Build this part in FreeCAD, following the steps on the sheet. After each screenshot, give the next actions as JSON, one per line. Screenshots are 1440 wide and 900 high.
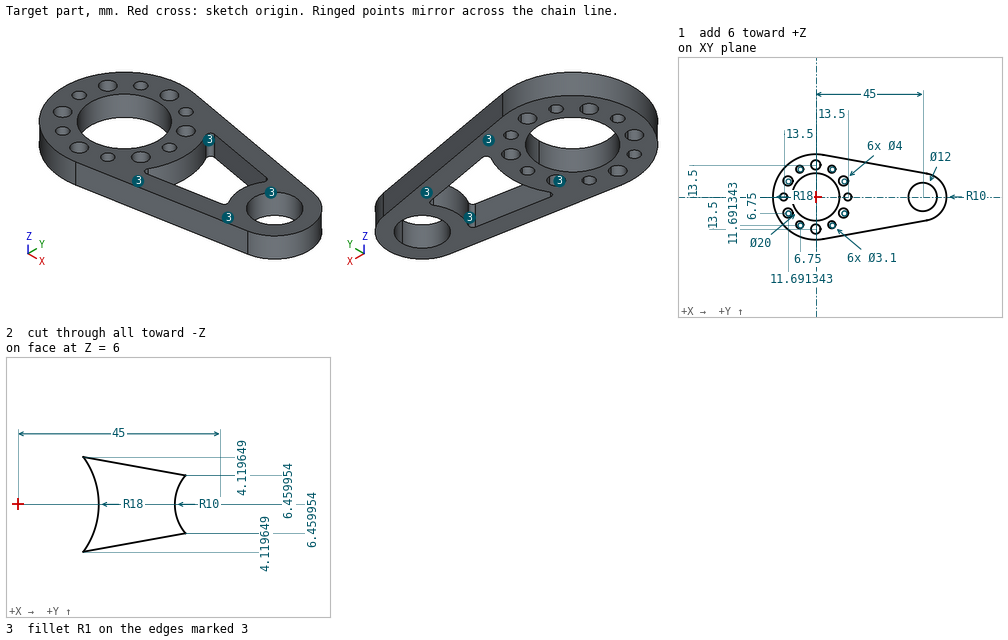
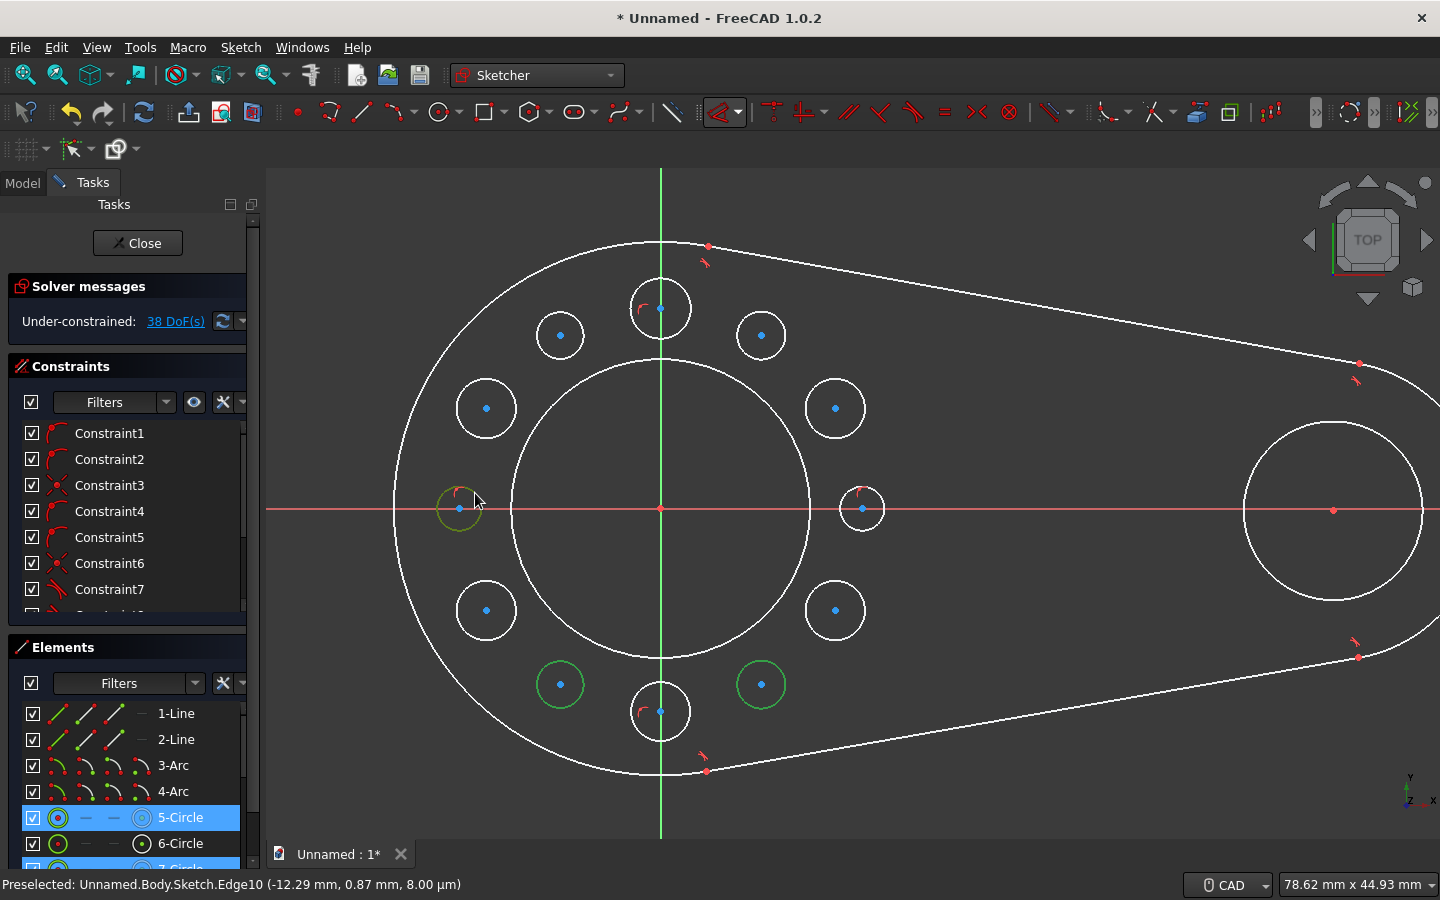
{"action": "left_click", "coordinate": [878, 493]}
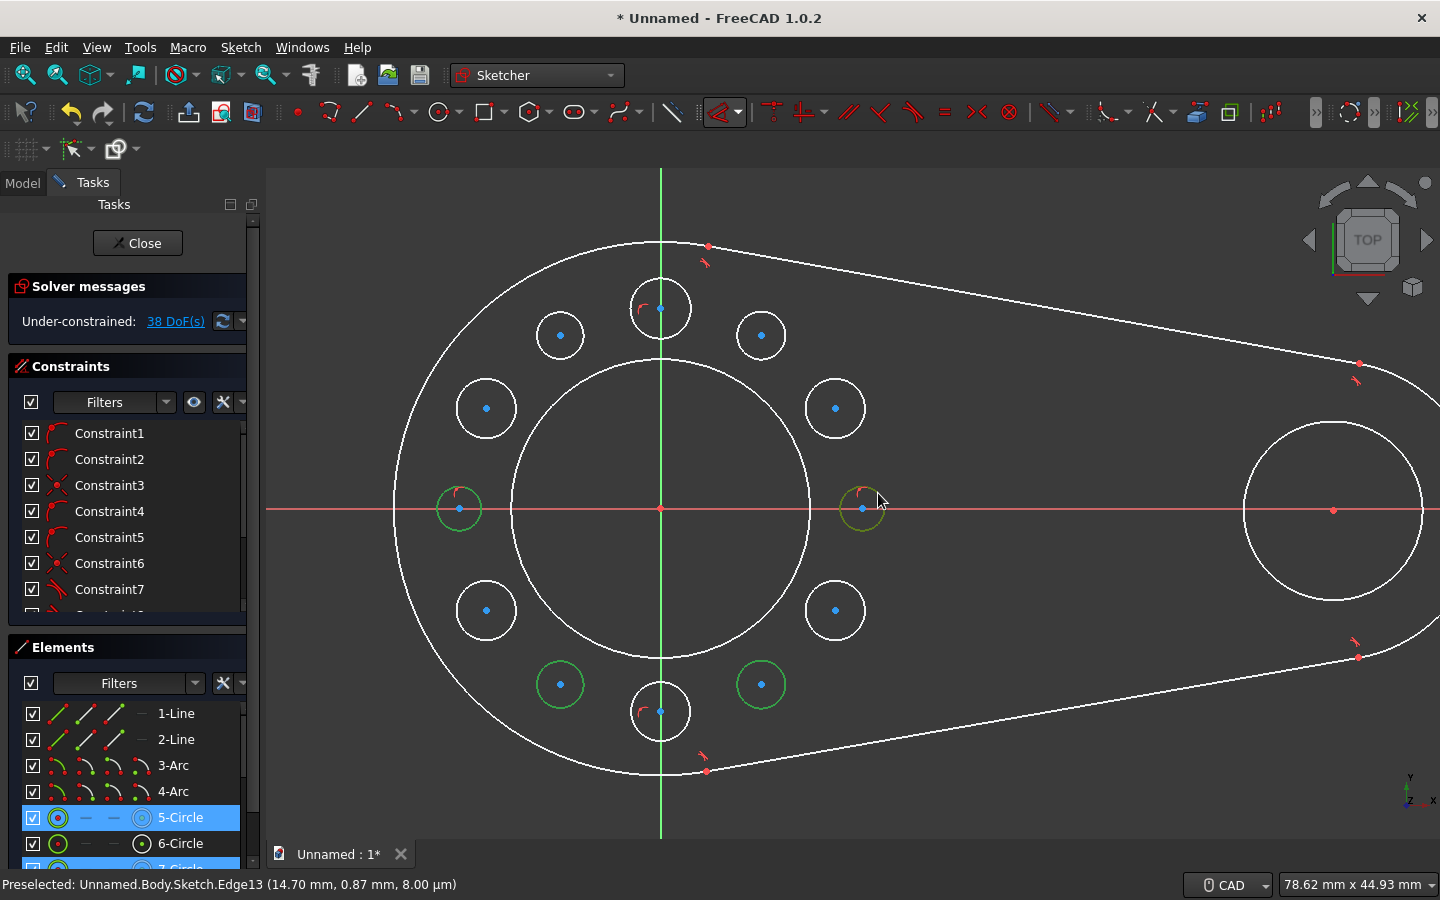
{"action": "left_click", "coordinate": [577, 319]}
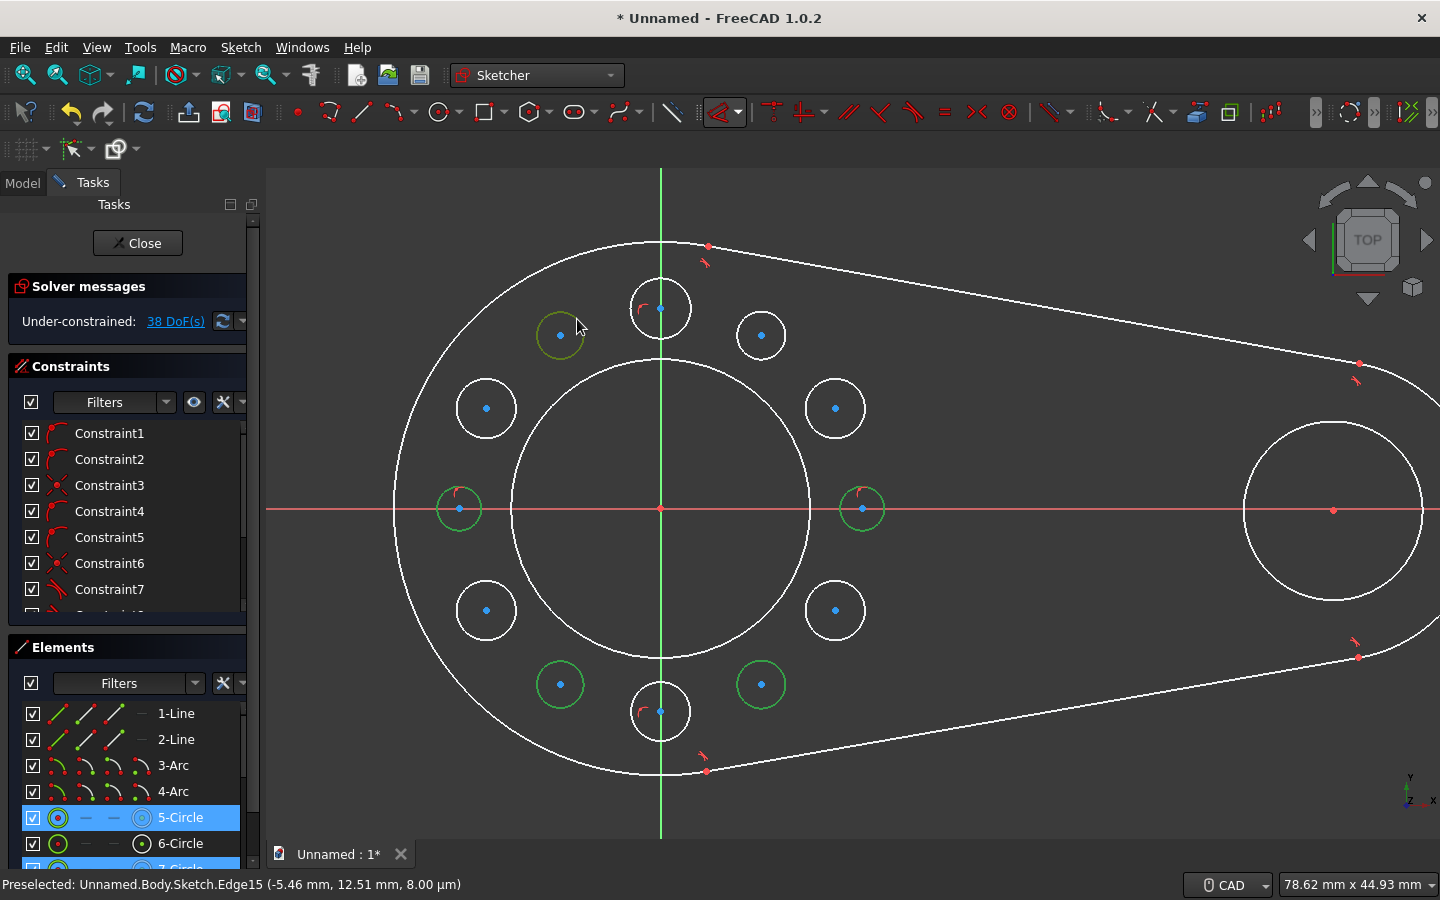
{"action": "left_click", "coordinate": [778, 318]}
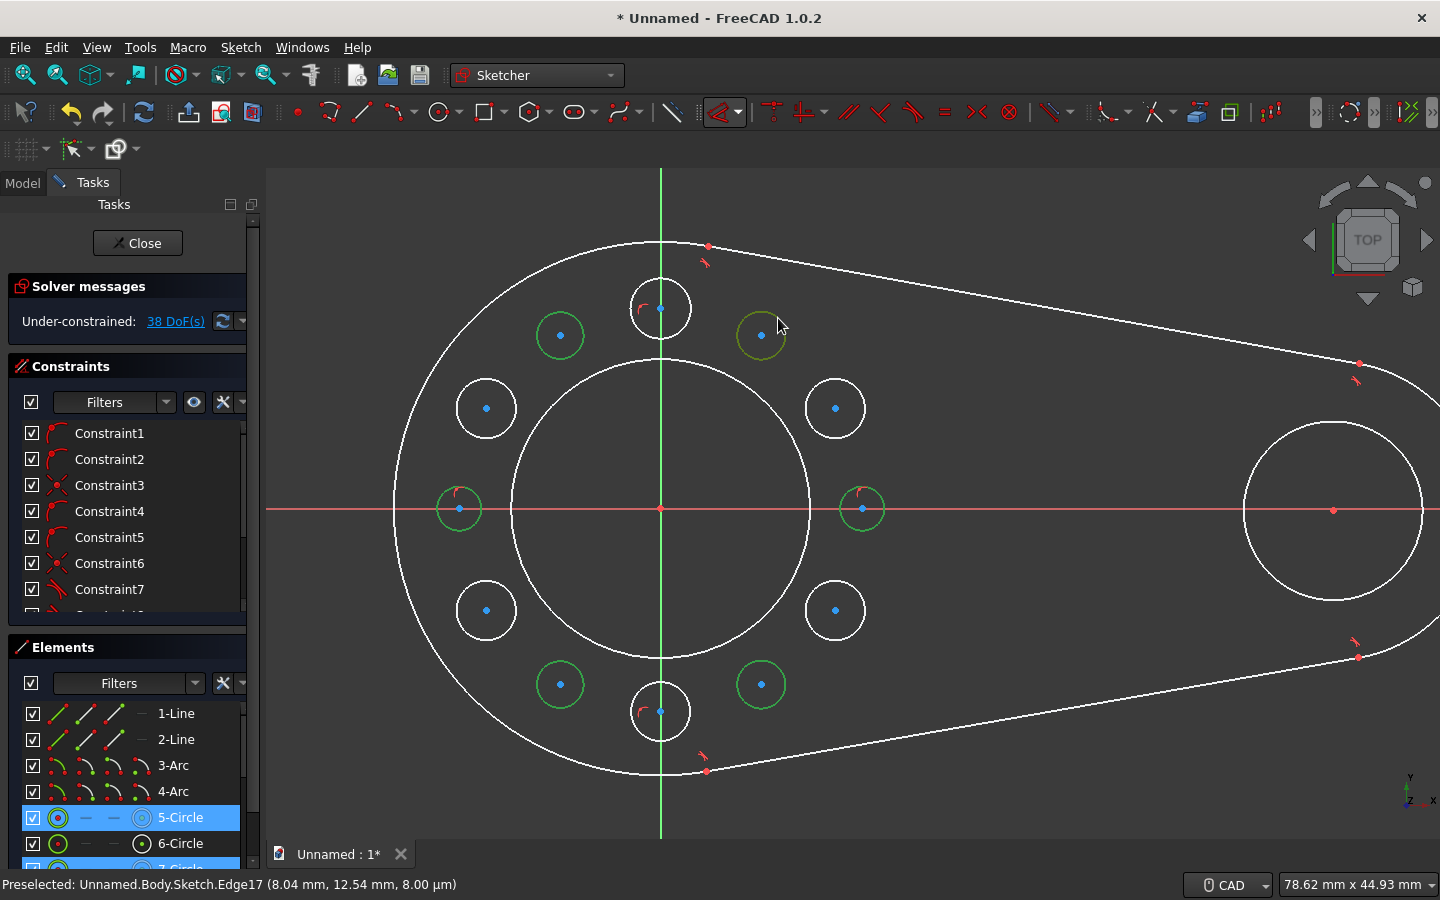
{"action": "key", "text": "e"}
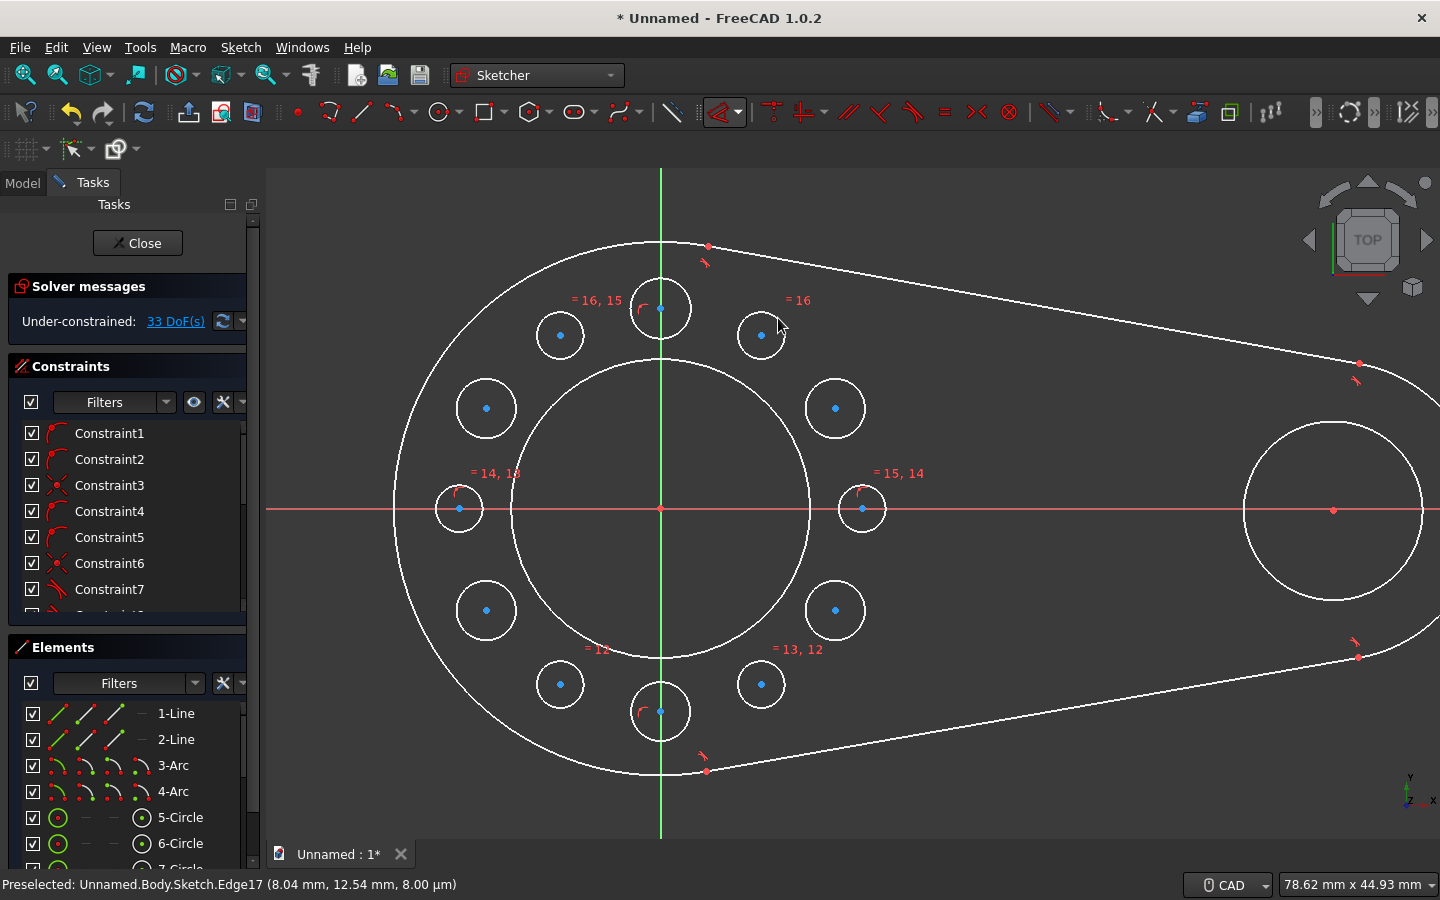
{"action": "left_click", "coordinate": [681, 691]}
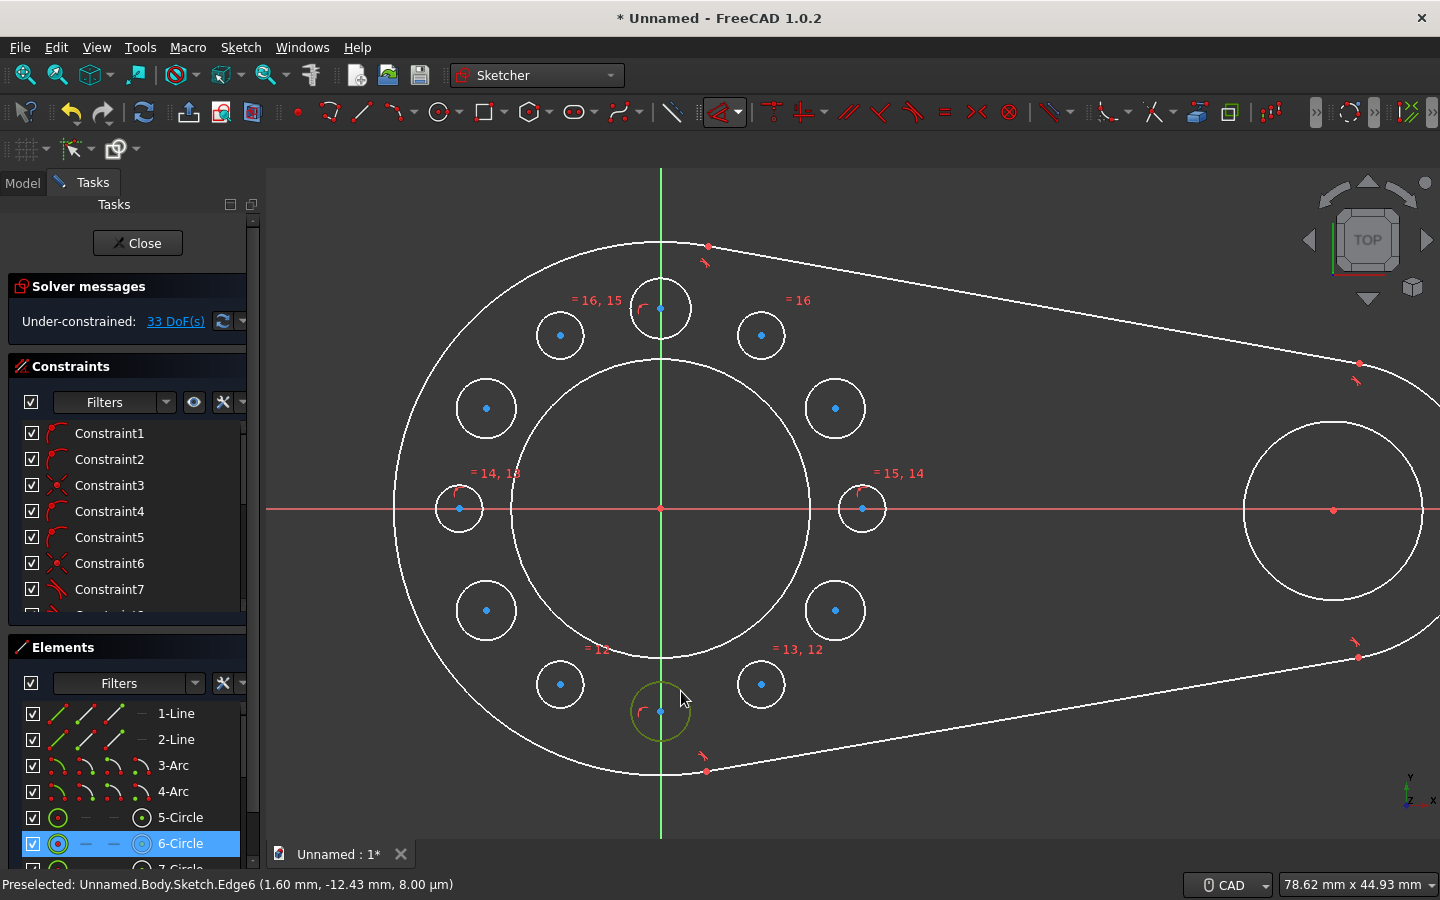
{"action": "left_click", "coordinate": [507, 589]}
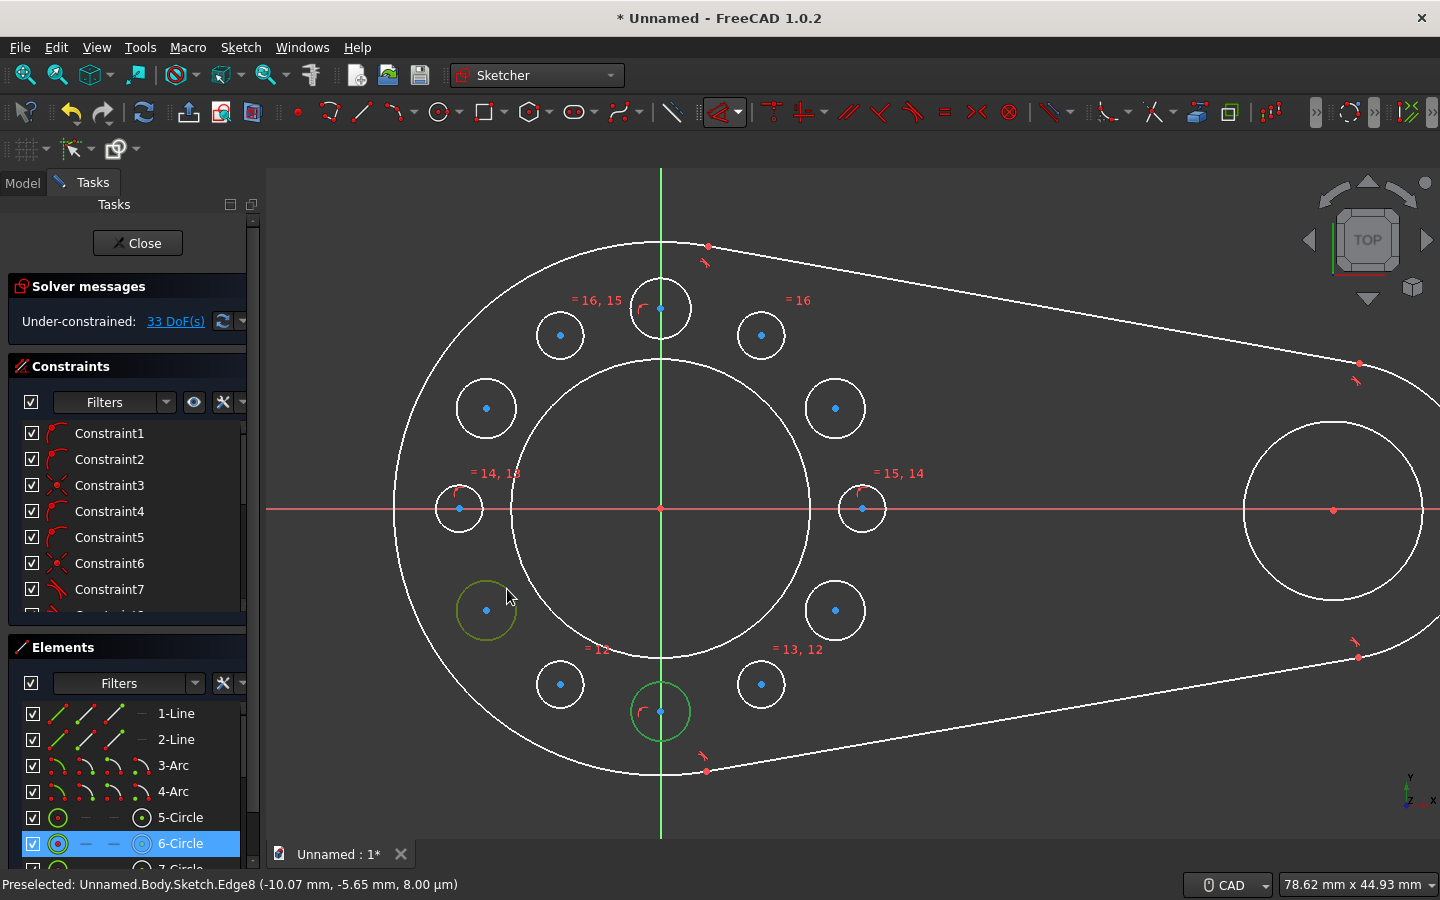
{"action": "left_click", "coordinate": [856, 589]}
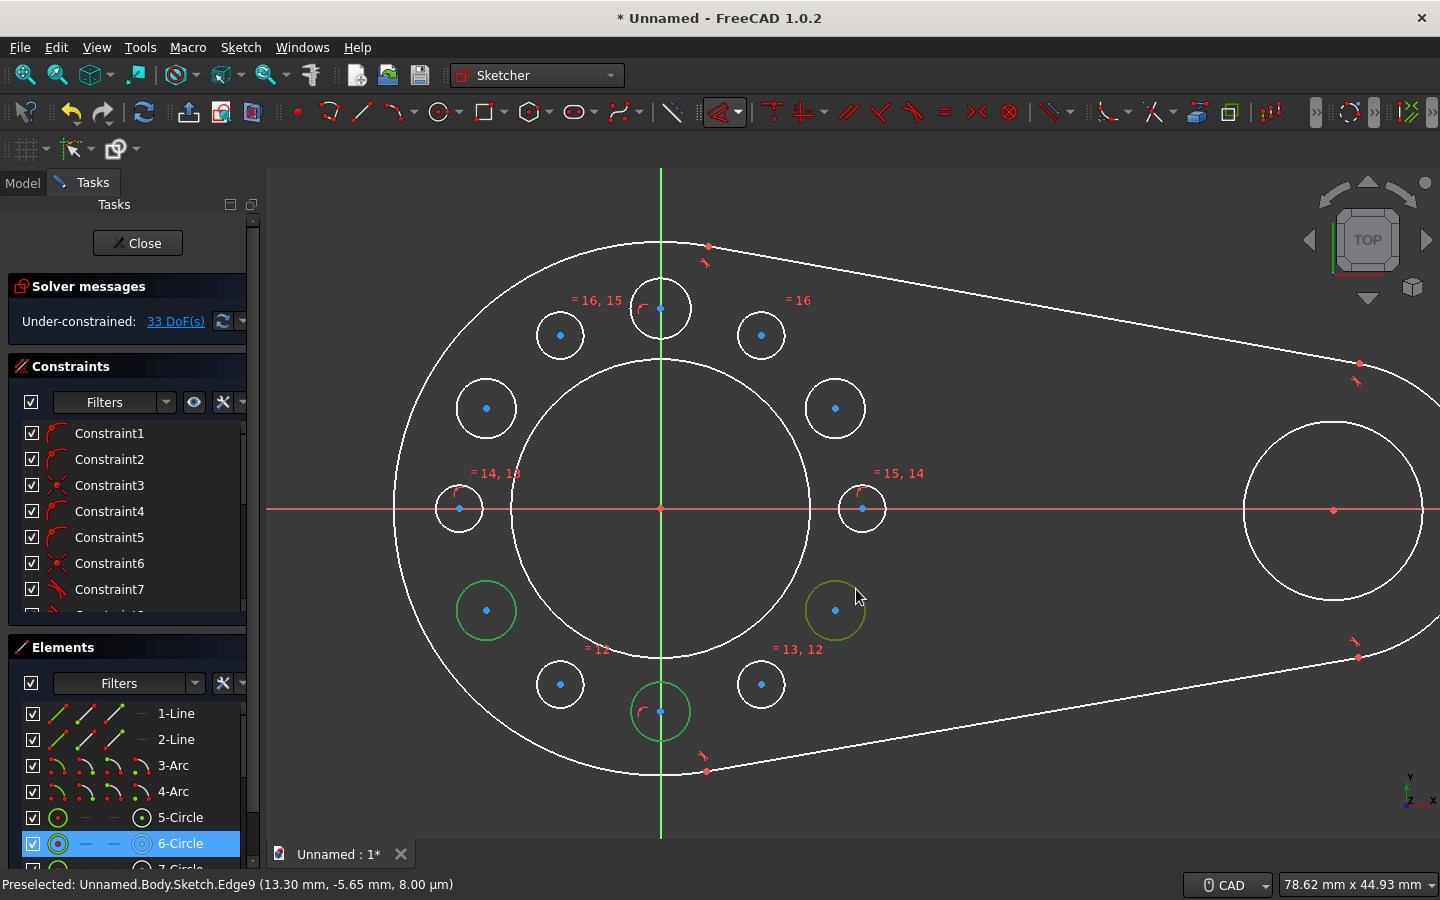
{"action": "left_click", "coordinate": [507, 387]}